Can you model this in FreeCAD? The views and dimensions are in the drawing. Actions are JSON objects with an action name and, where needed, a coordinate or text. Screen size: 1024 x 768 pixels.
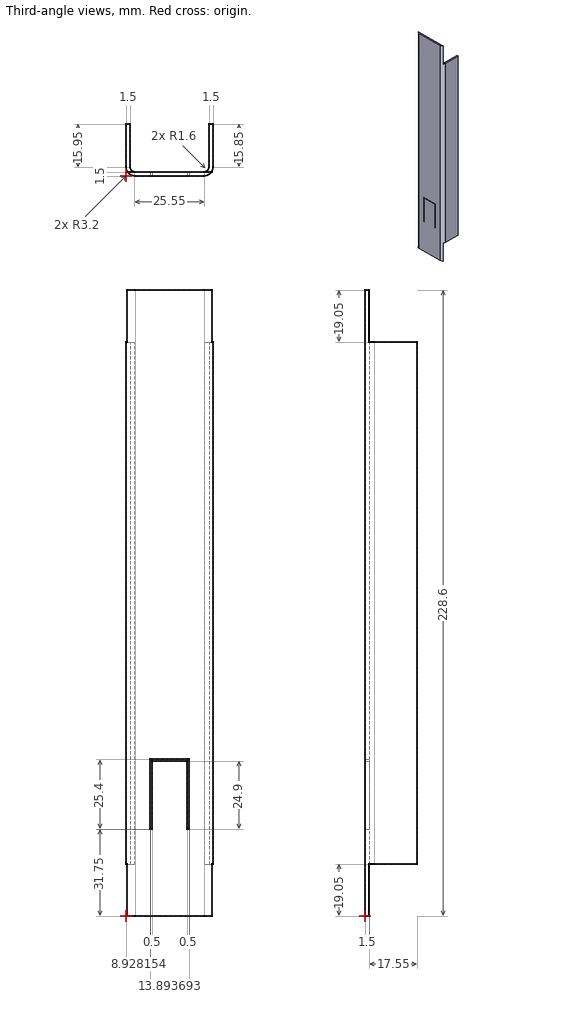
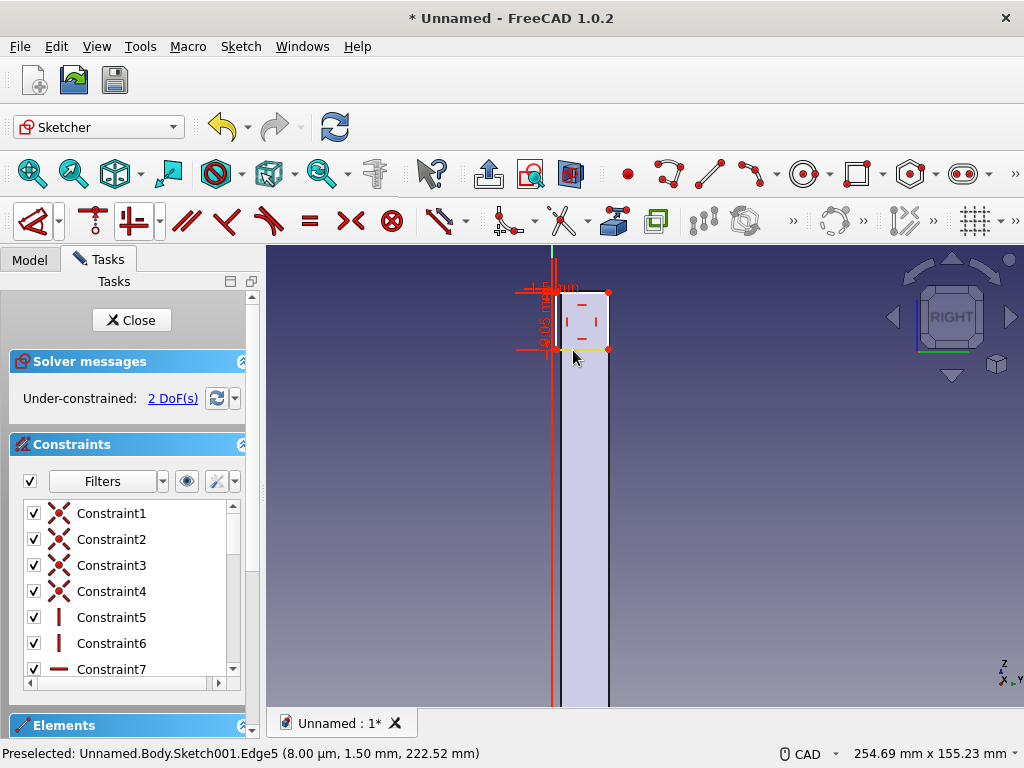
{"action": "left_click", "coordinate": [572, 350]}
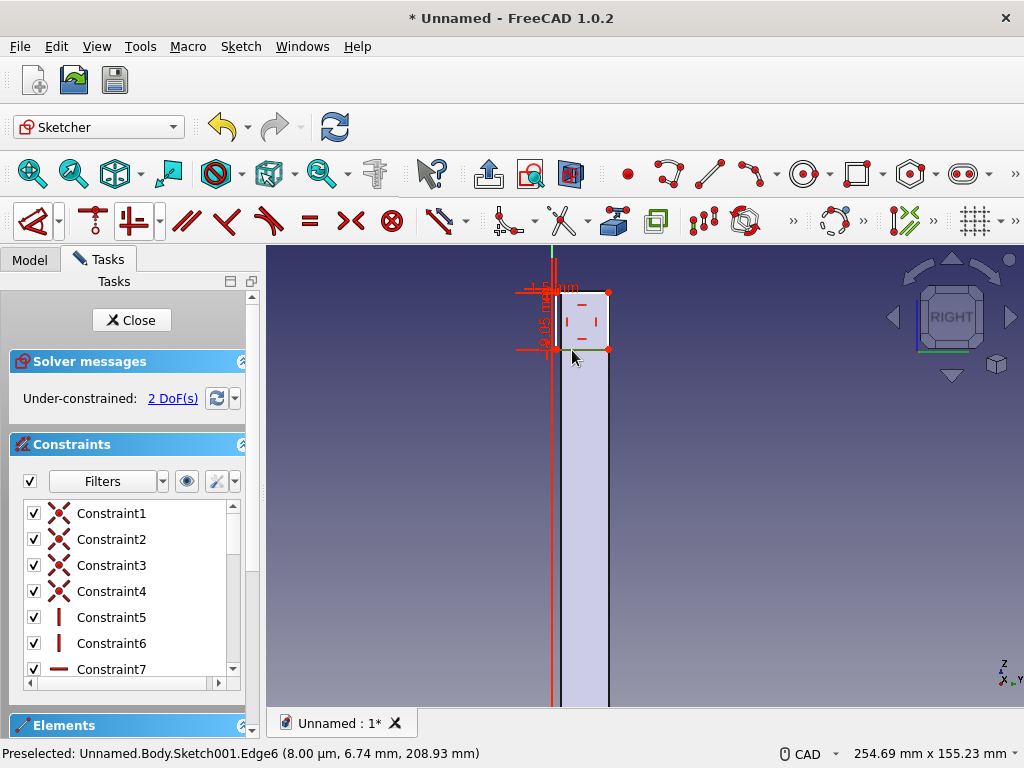
{"action": "key", "text": "l"}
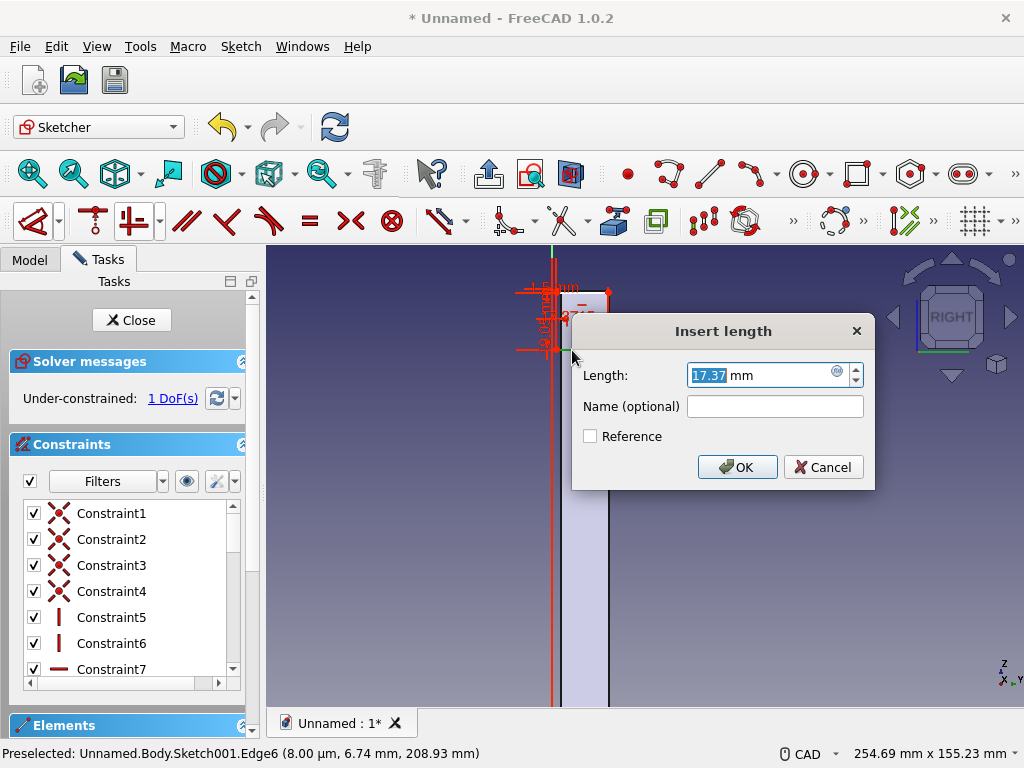
{"action": "type", "text": "17.55"}
{"action": "key", "text": "Return"}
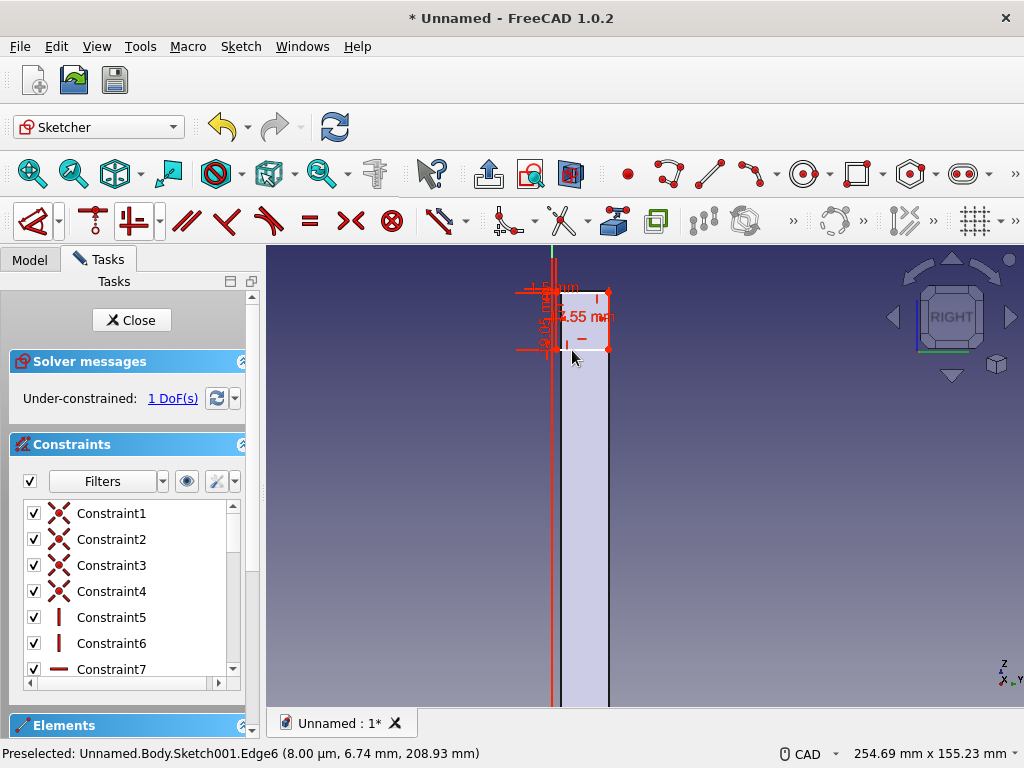
{"action": "left_click", "coordinate": [556, 293]}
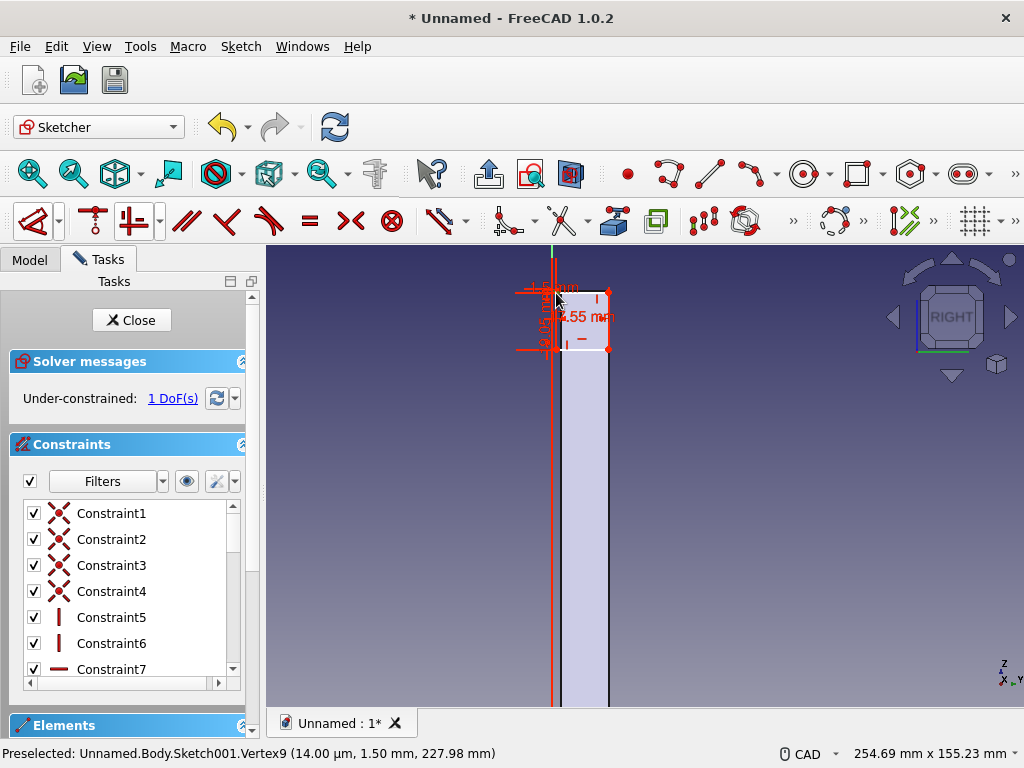
{"action": "left_click", "coordinate": [58, 222]}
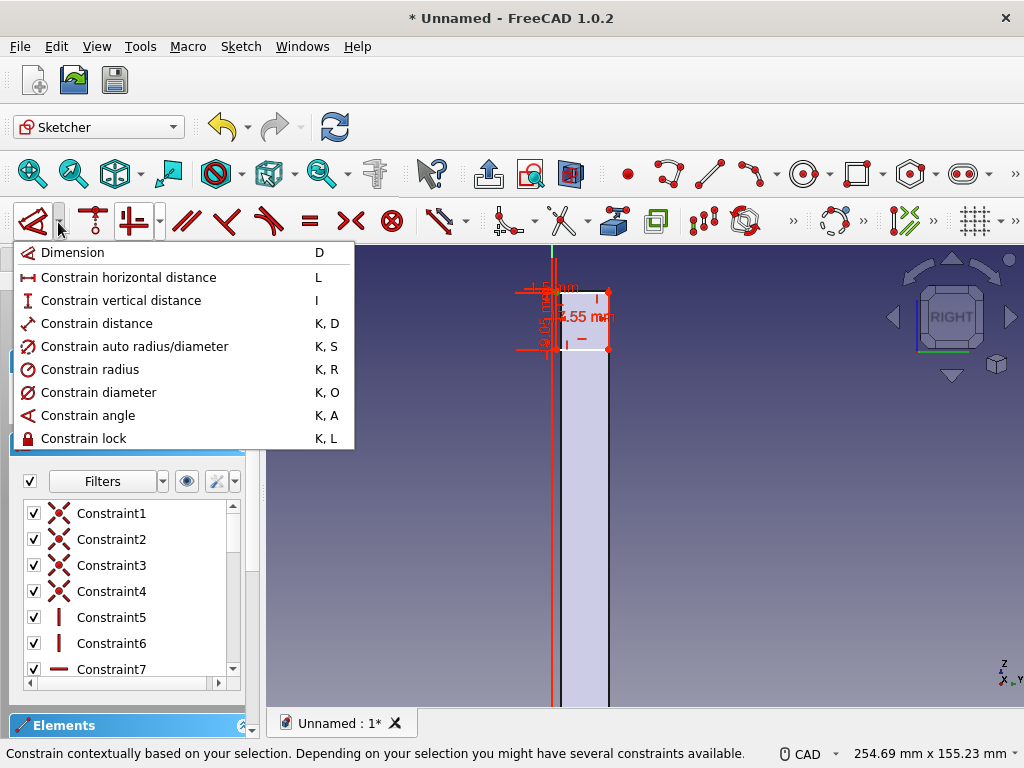
{"action": "left_click", "coordinate": [184, 300]}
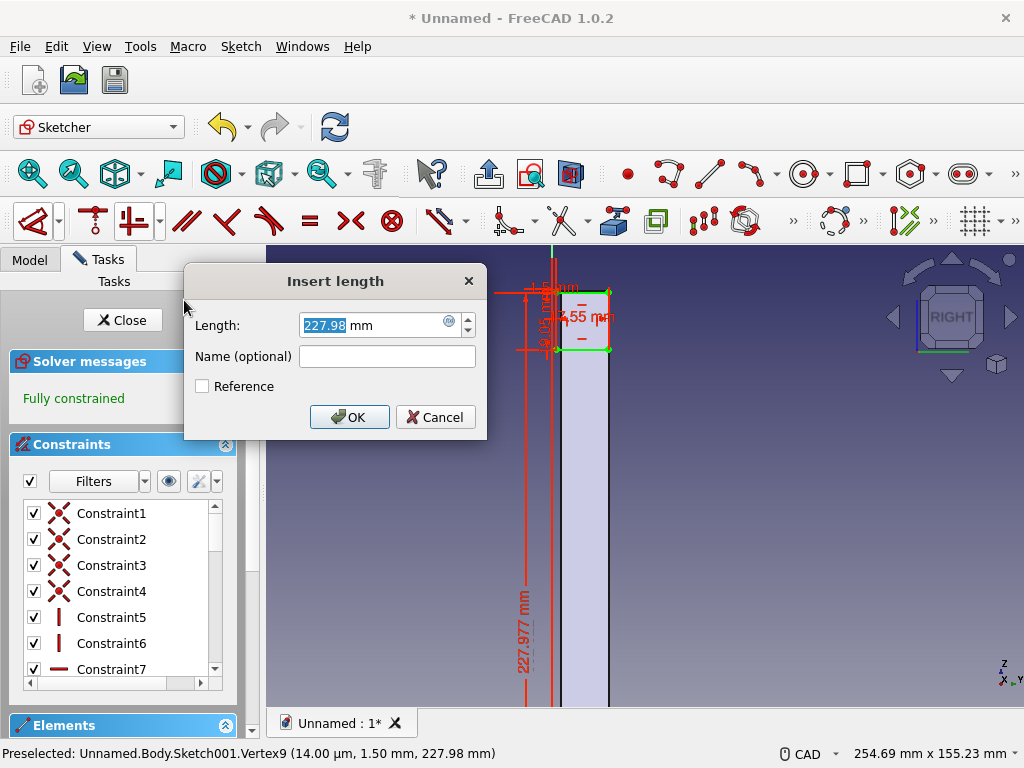
{"action": "type", "text": "228.6"}
{"action": "key", "text": "Return"}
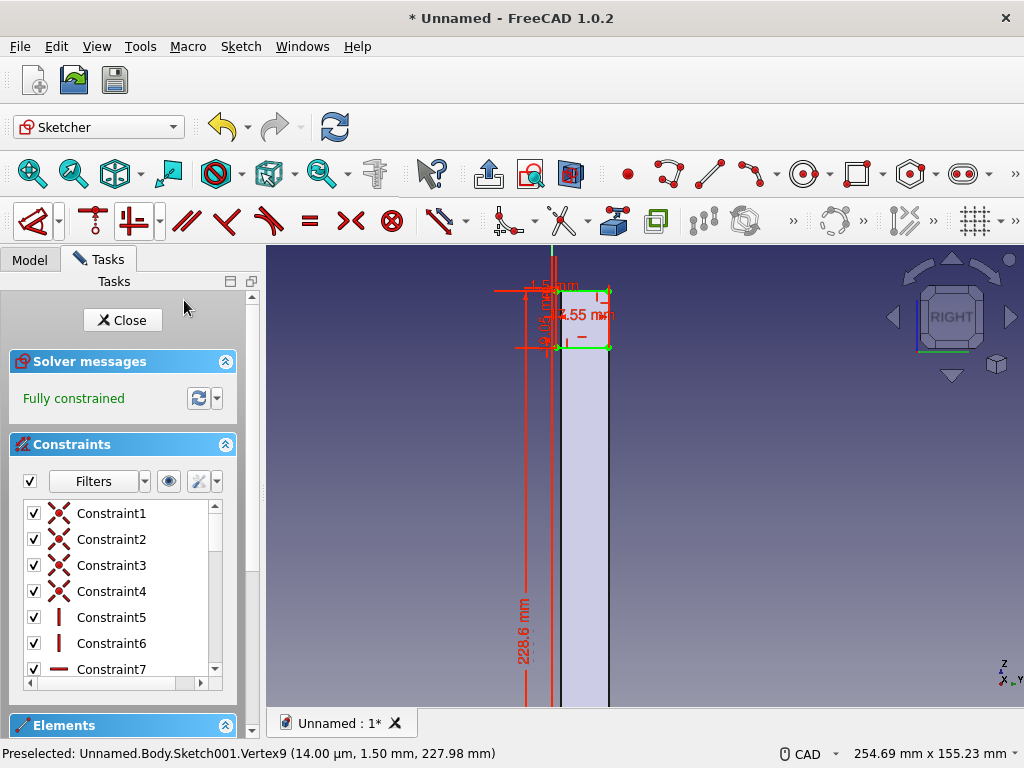
{"action": "left_click", "coordinate": [123, 320]}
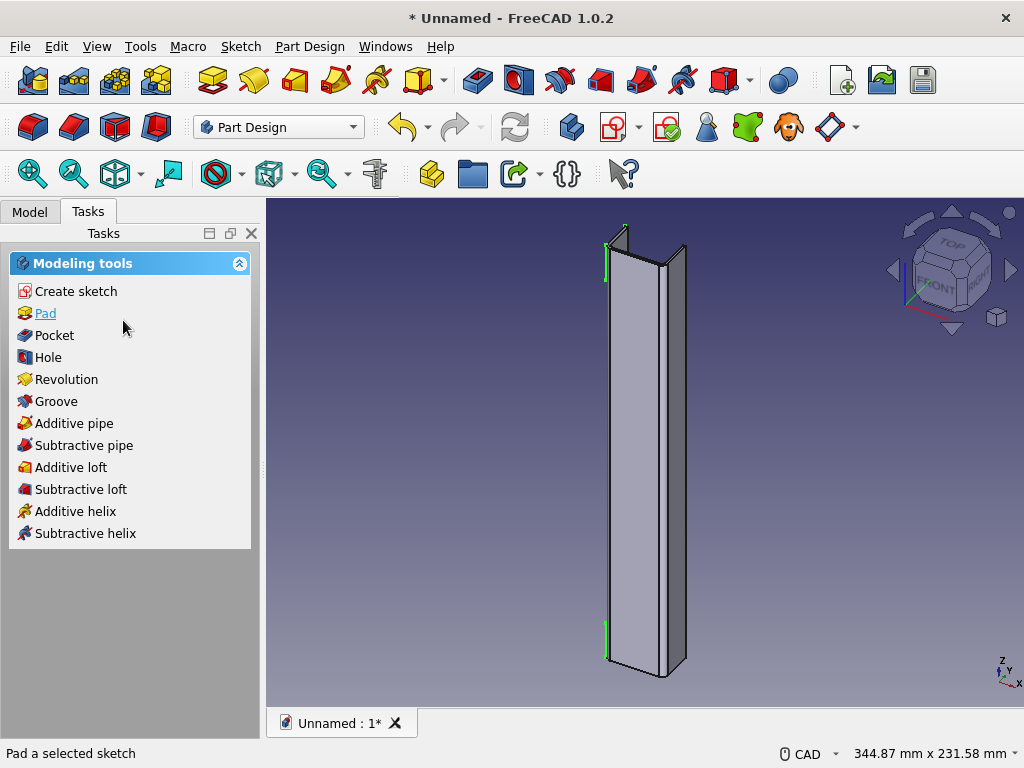
{"action": "left_click", "coordinate": [478, 80]}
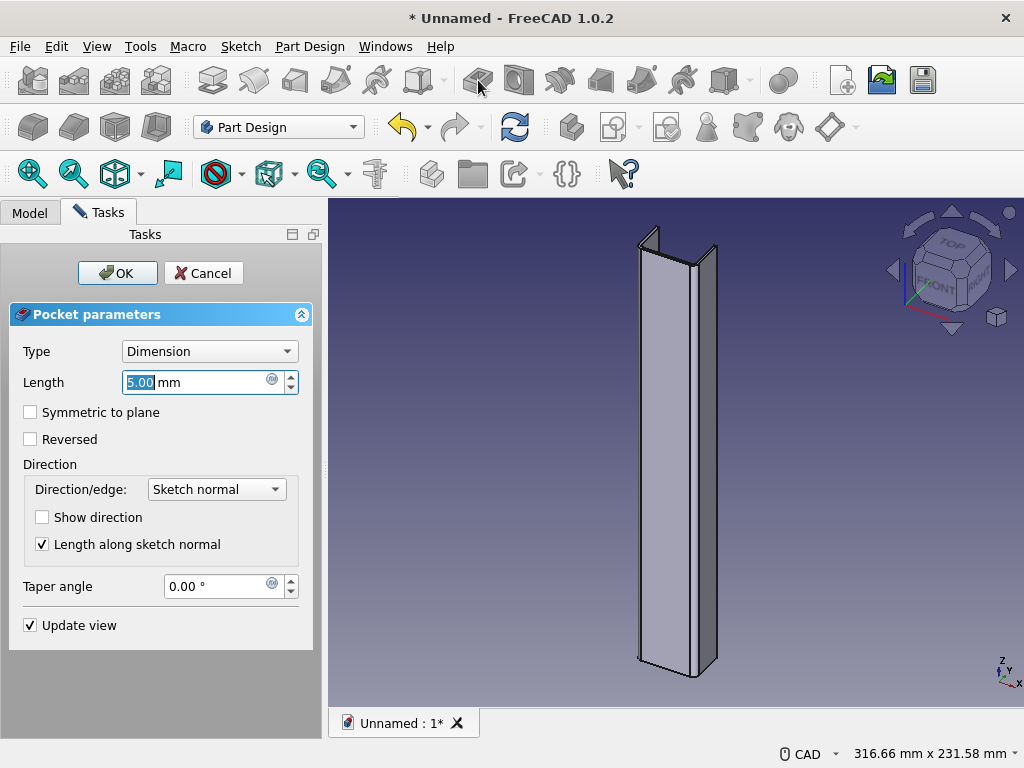
{"action": "left_click", "coordinate": [210, 352]}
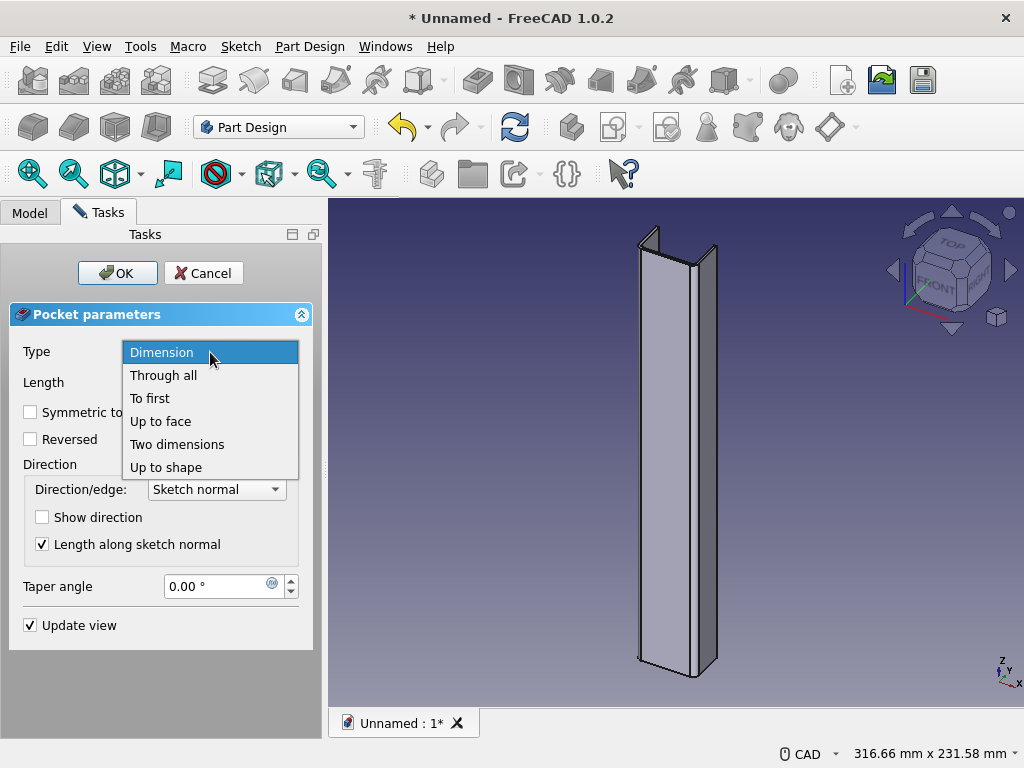
{"action": "left_click", "coordinate": [208, 376]}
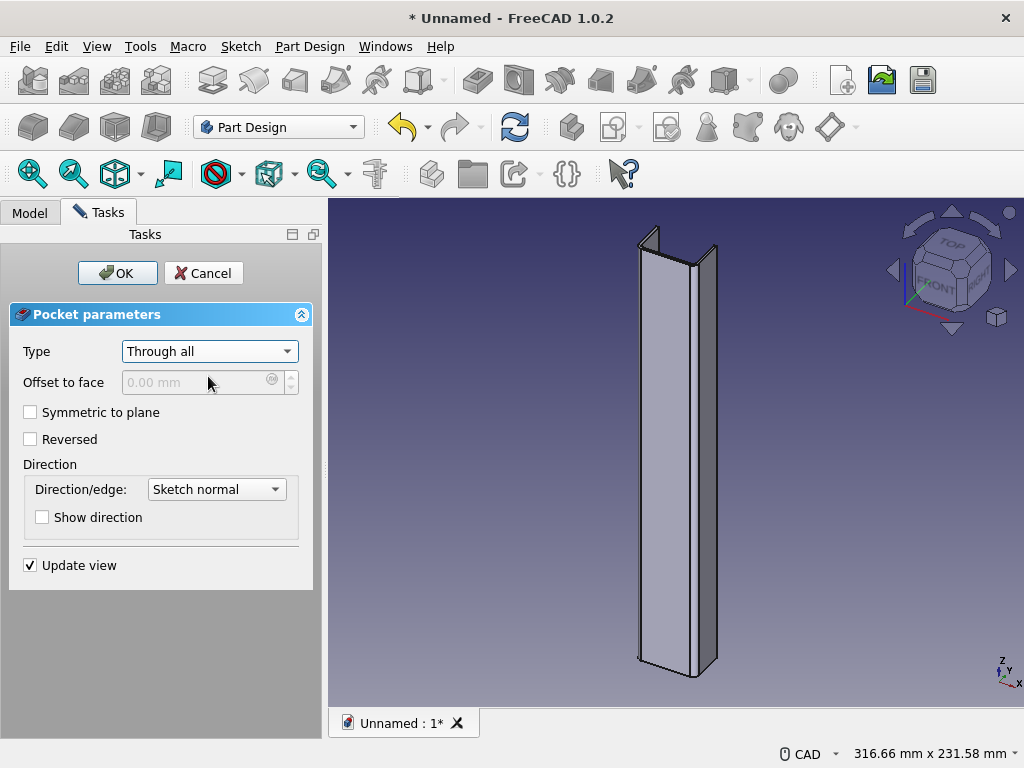
{"action": "left_click", "coordinate": [31, 439]}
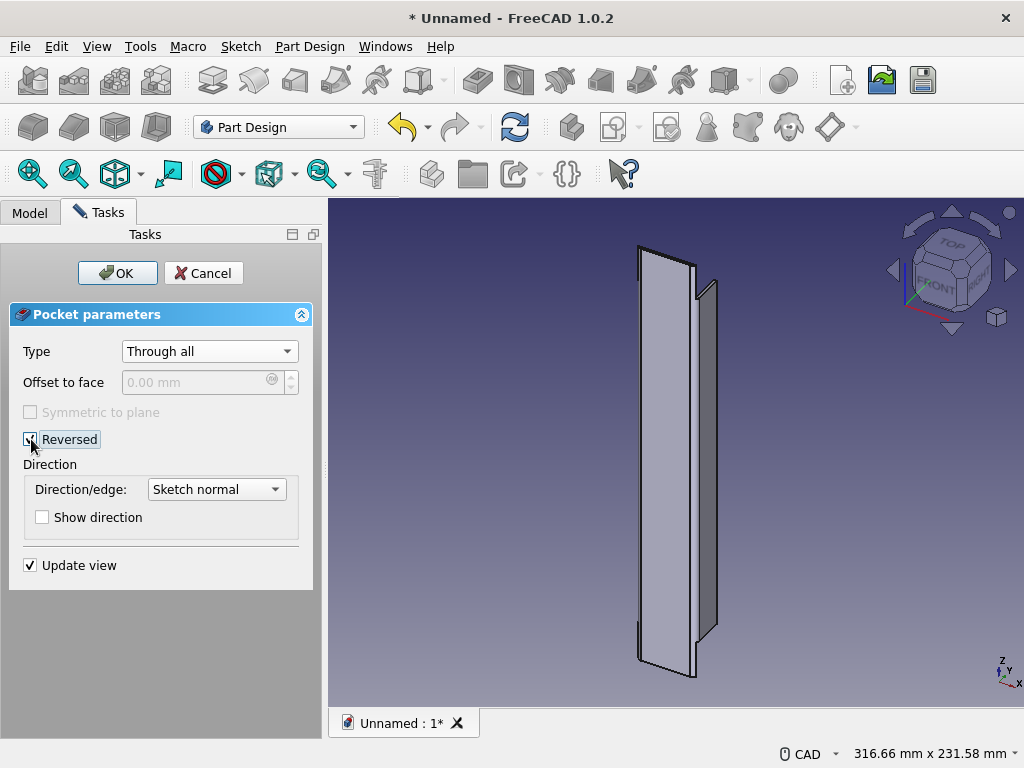
{"action": "left_click", "coordinate": [118, 273]}